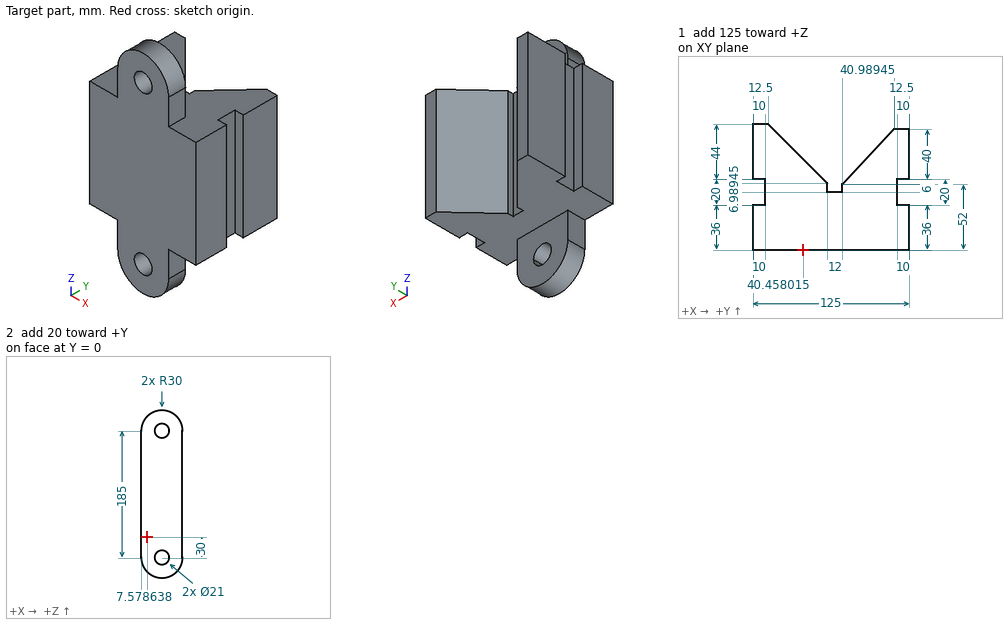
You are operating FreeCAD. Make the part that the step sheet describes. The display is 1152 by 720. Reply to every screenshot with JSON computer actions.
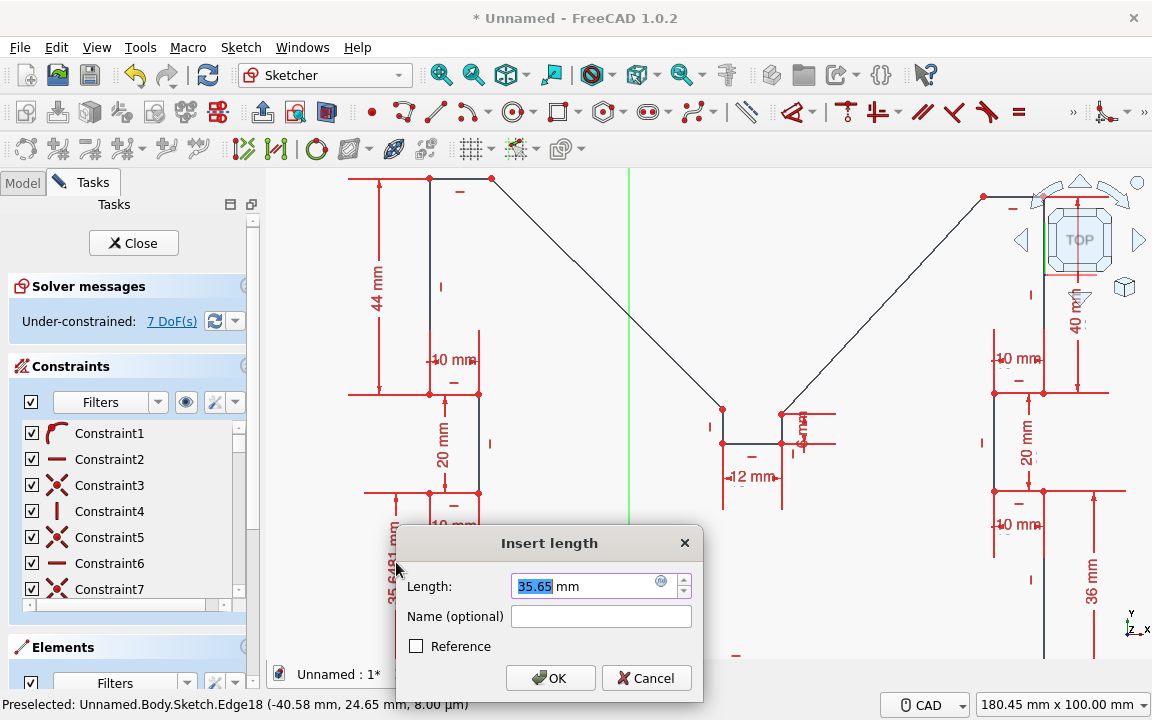
{"action": "type", "text": "36"}
{"action": "key", "text": "Return"}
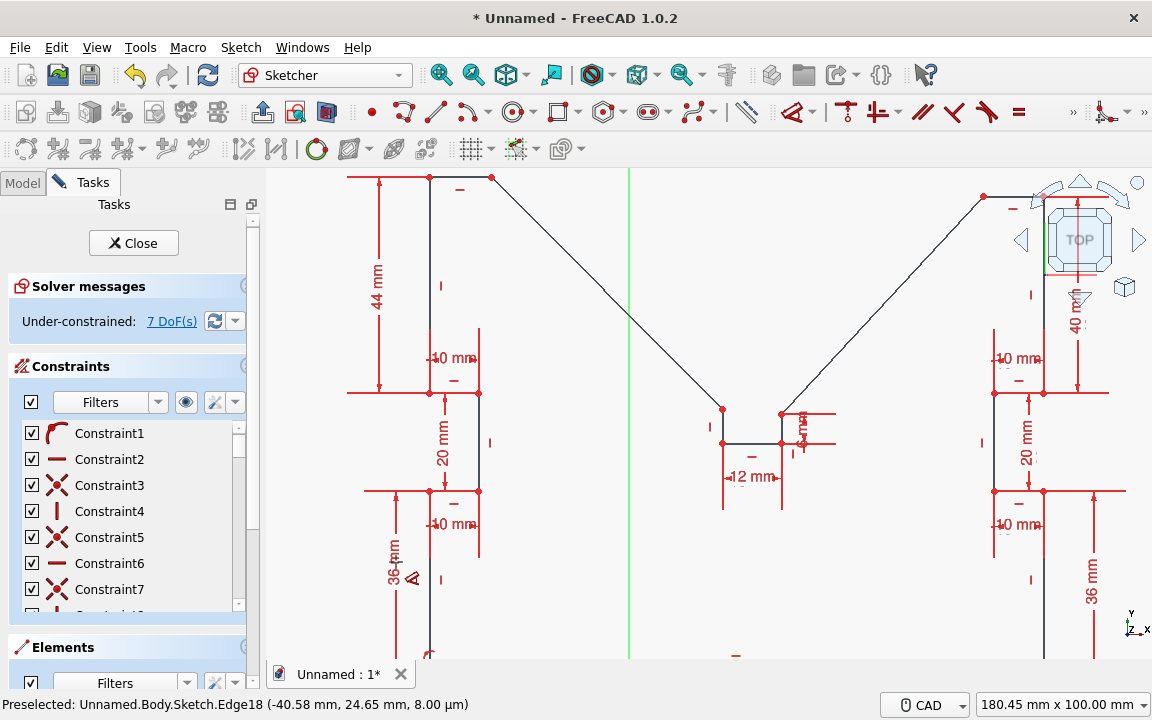
{"action": "scroll", "coordinate": [444, 395], "scroll_direction": "down", "scroll_amount": 2}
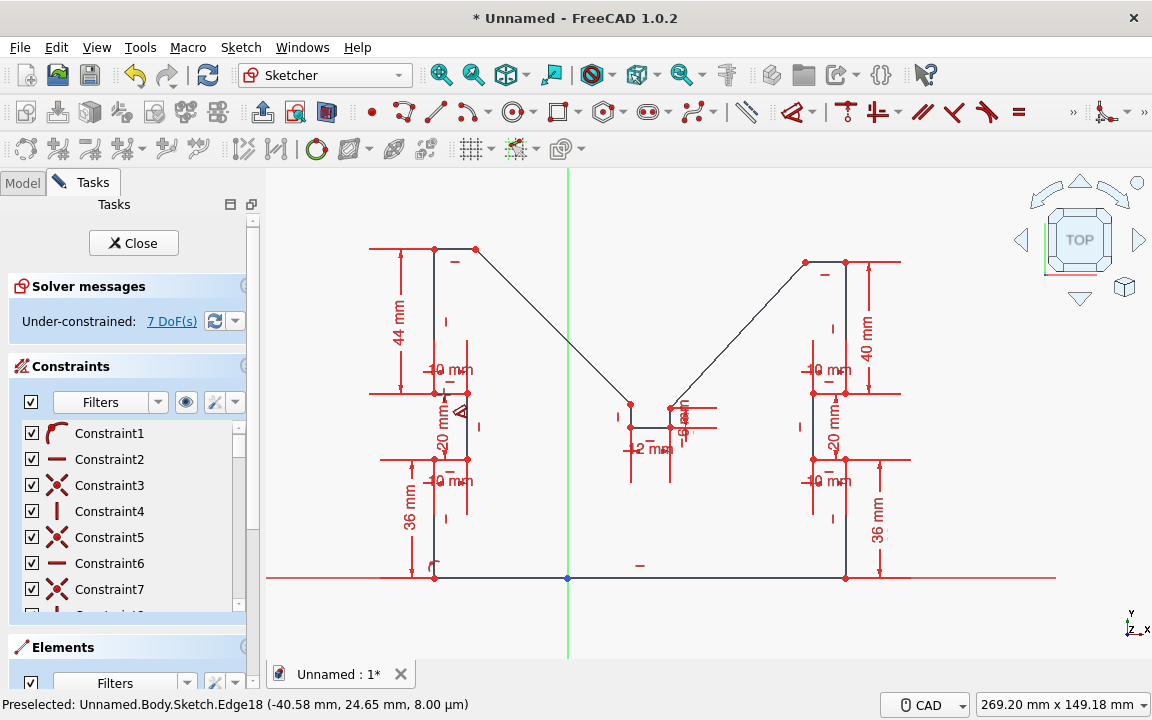
{"action": "scroll", "coordinate": [558, 578], "scroll_direction": "up", "scroll_amount": 2}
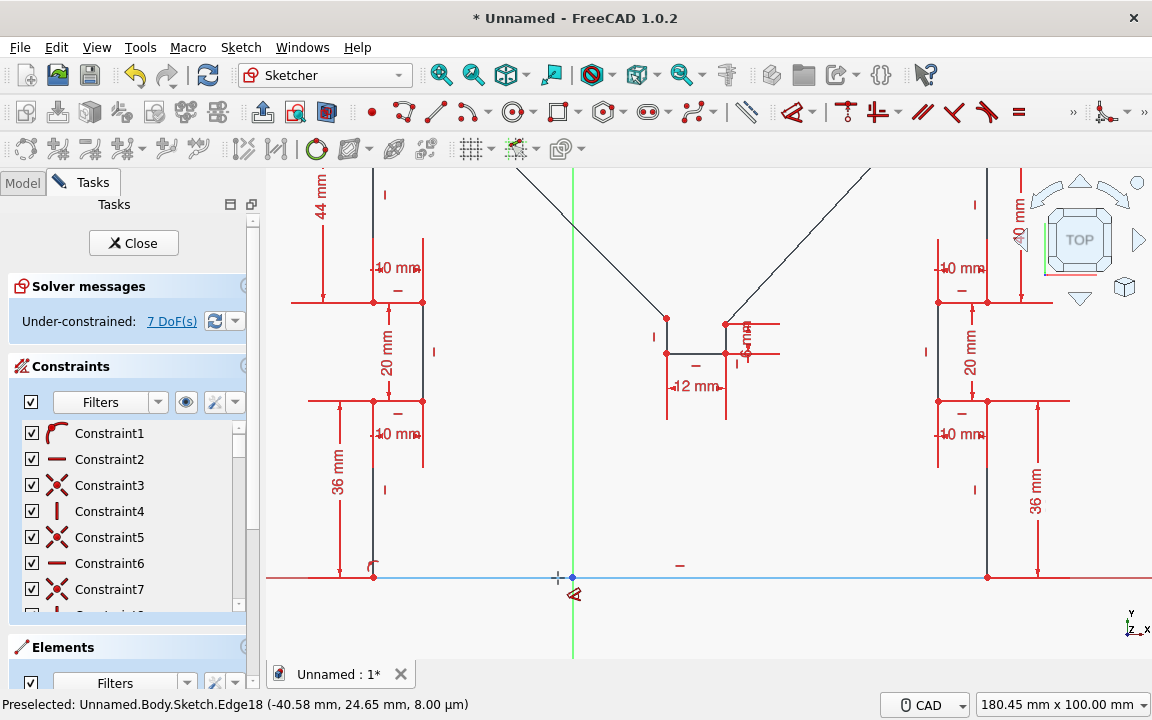
{"action": "left_click", "coordinate": [558, 578]}
{"action": "left_click", "coordinate": [680, 612]}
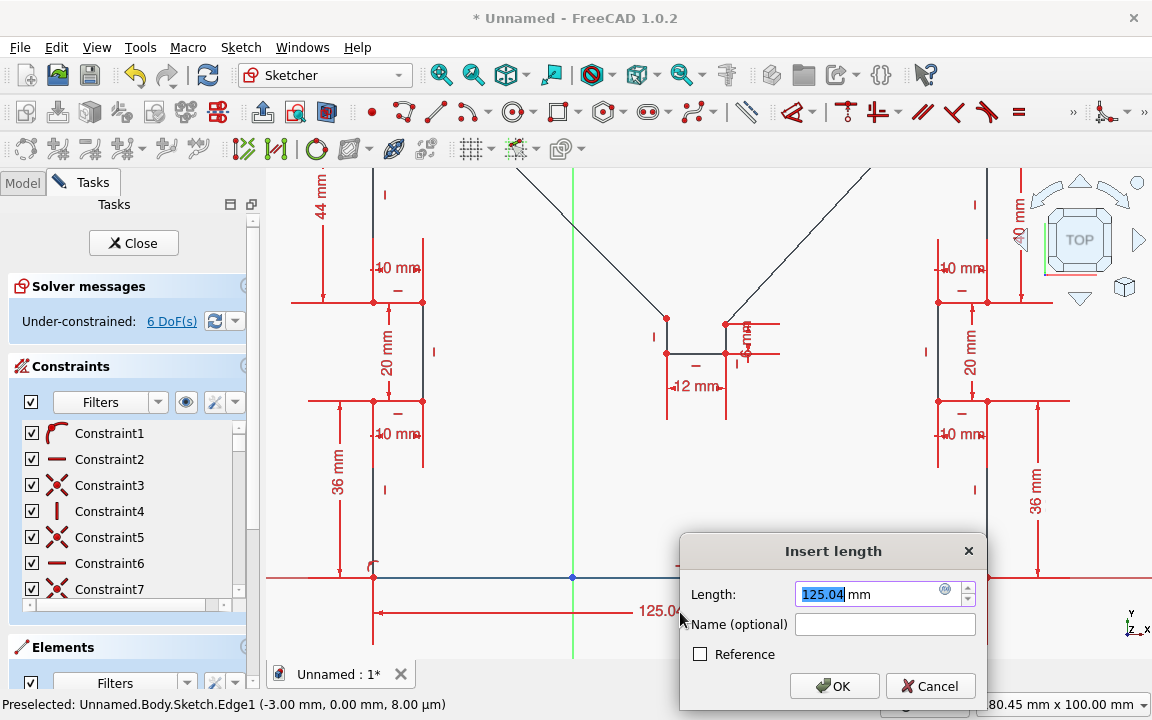
{"action": "type", "text": "125"}
{"action": "key", "text": "Return"}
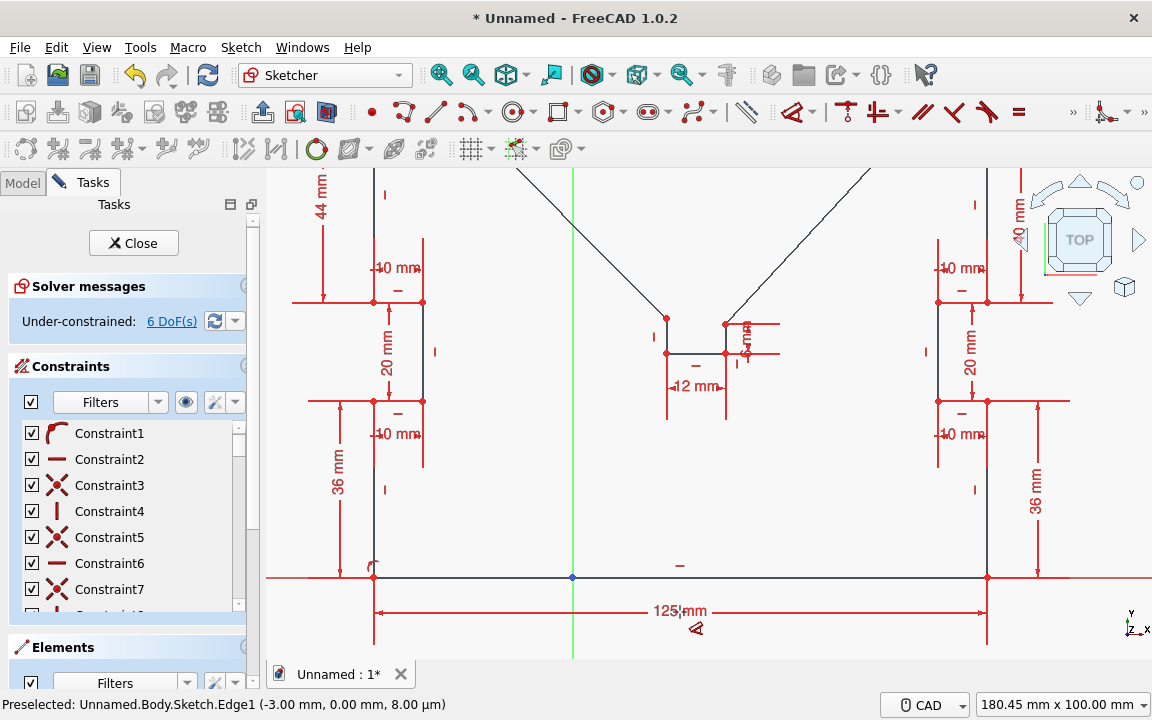
{"action": "left_click", "coordinate": [726, 324]}
{"action": "left_click", "coordinate": [539, 451]}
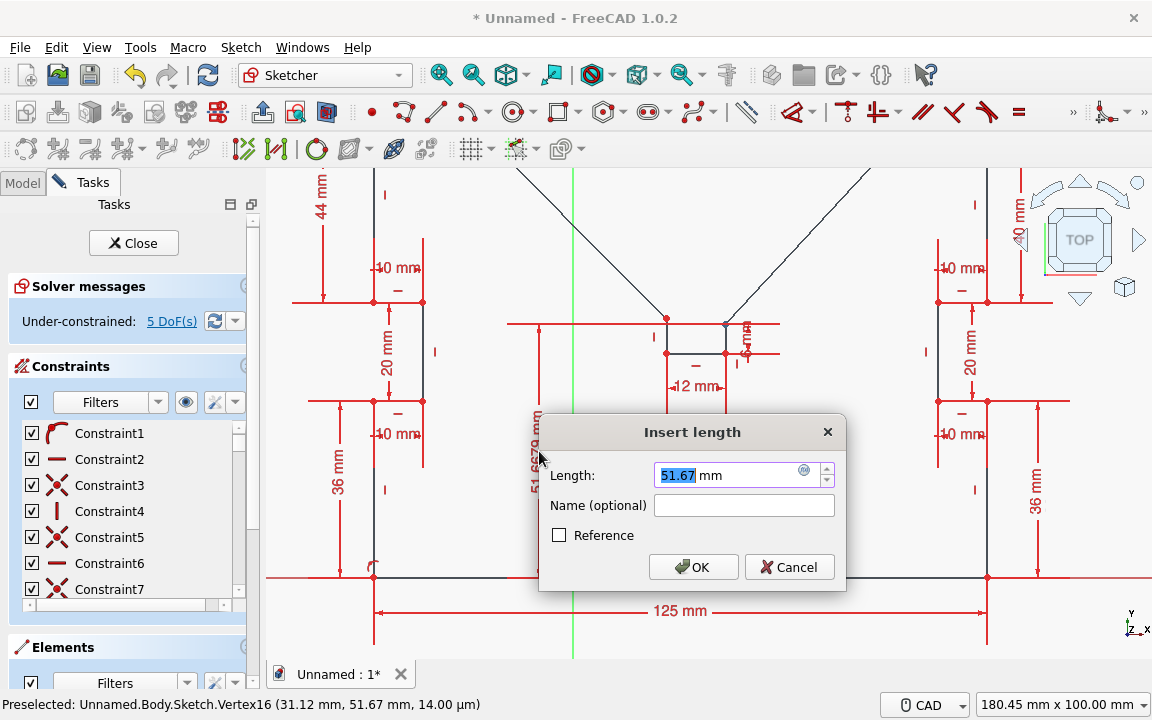
{"action": "type", "text": "52"}
{"action": "key", "text": "Return"}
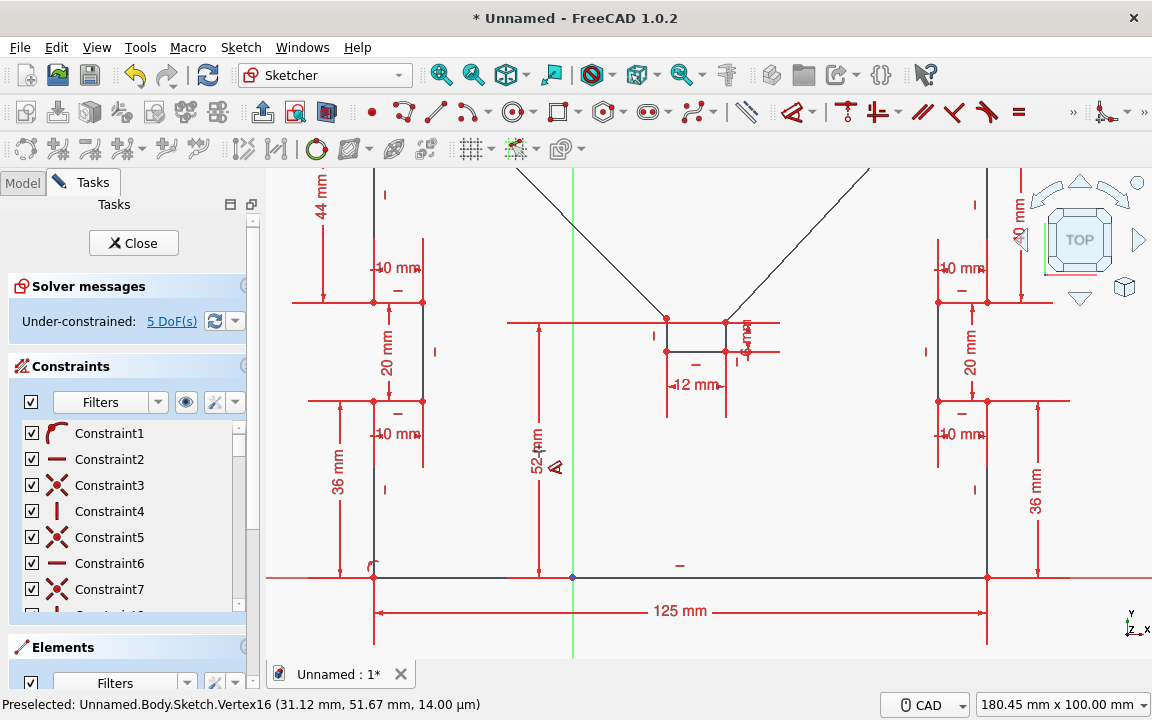
{"action": "scroll", "coordinate": [558, 579], "scroll_direction": "down", "scroll_amount": 2}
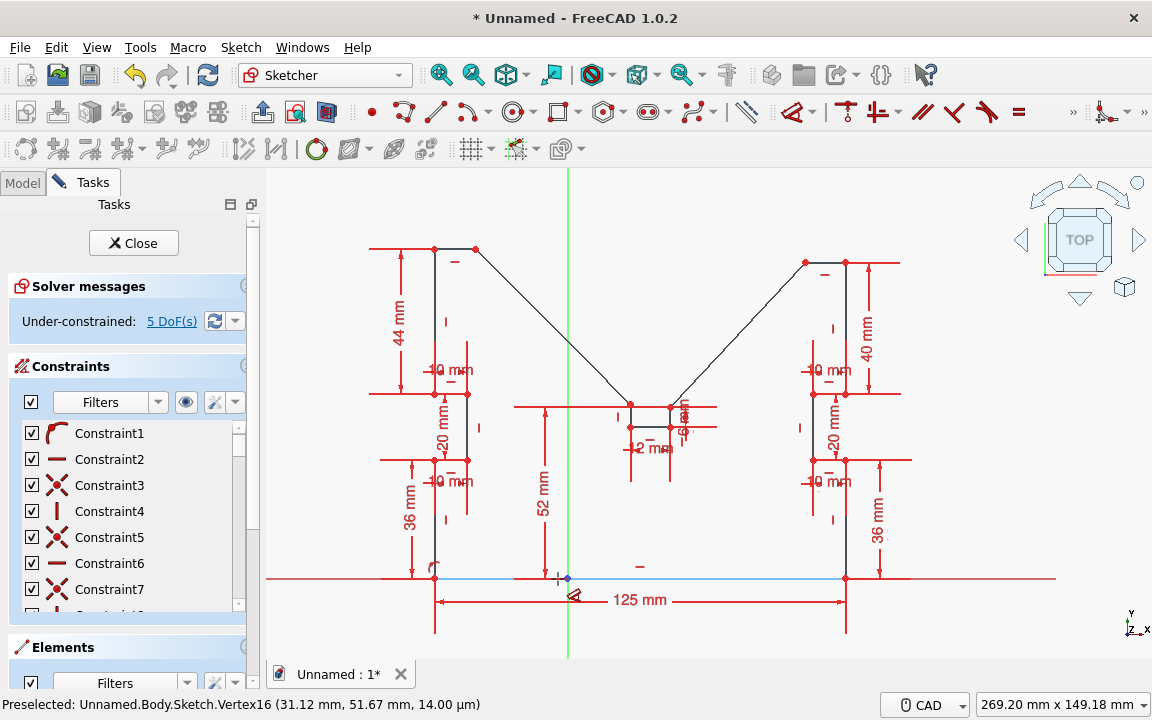
{"action": "left_click", "coordinate": [834, 263]}
{"action": "left_click", "coordinate": [826, 229]}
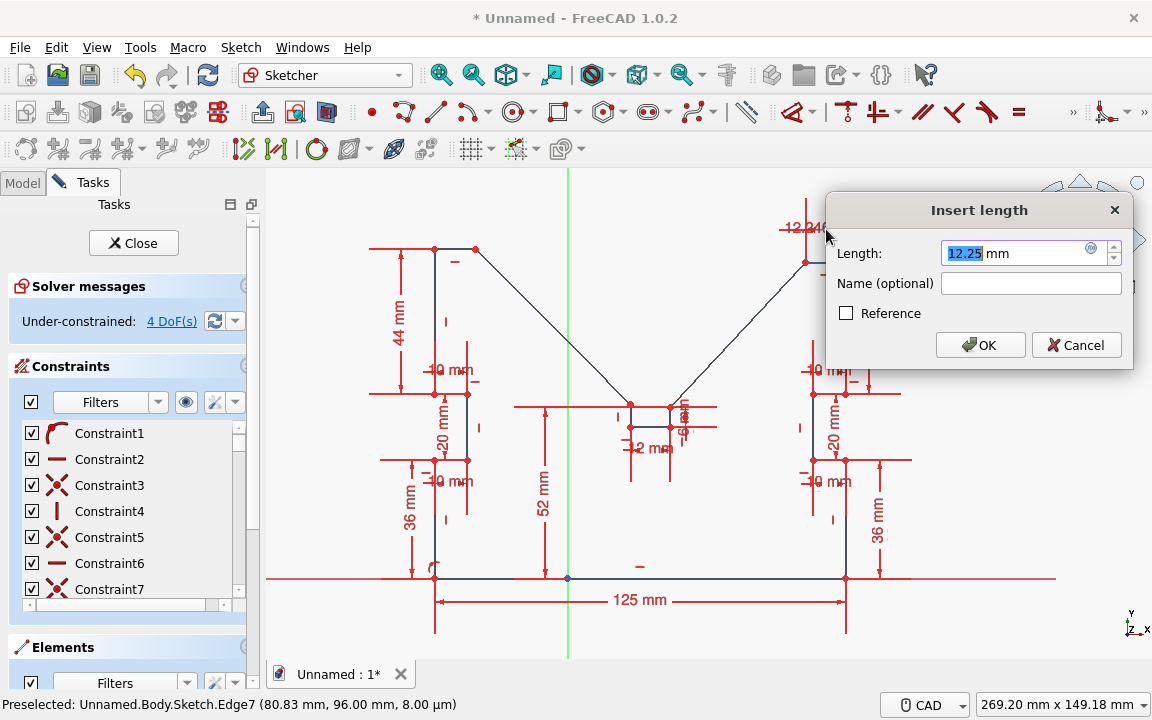
{"action": "type", "text": "12.5"}
{"action": "key", "text": "Return"}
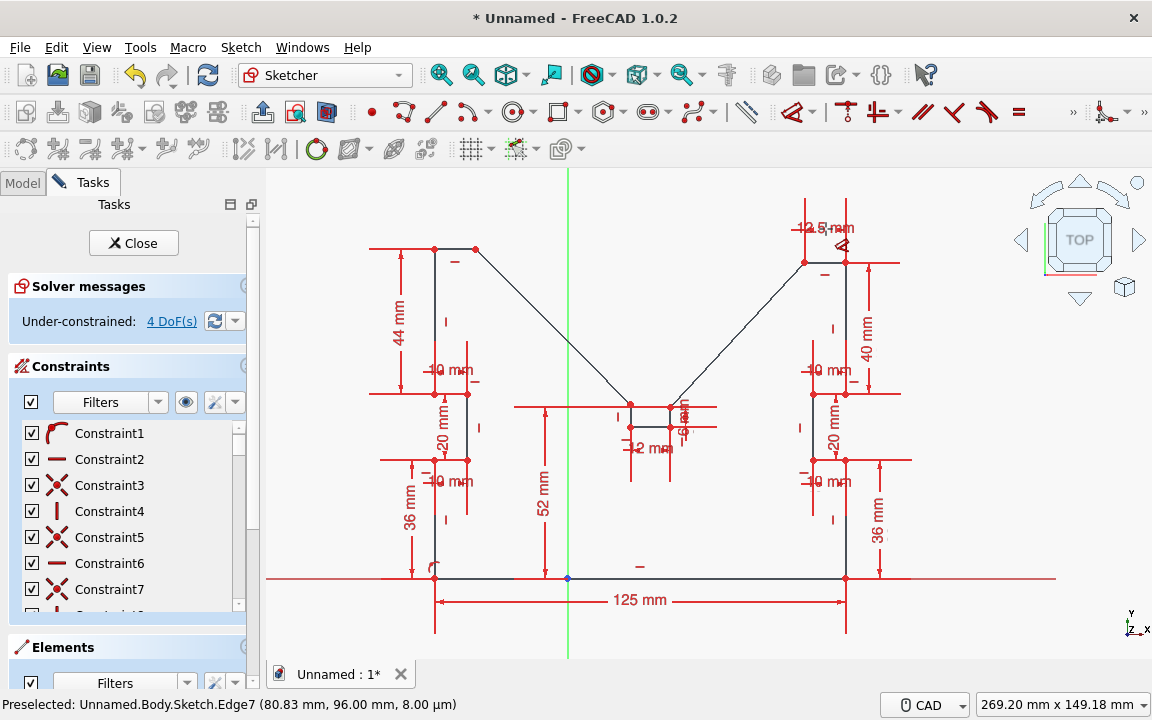
{"action": "left_click", "coordinate": [463, 249]}
{"action": "left_click", "coordinate": [455, 215]}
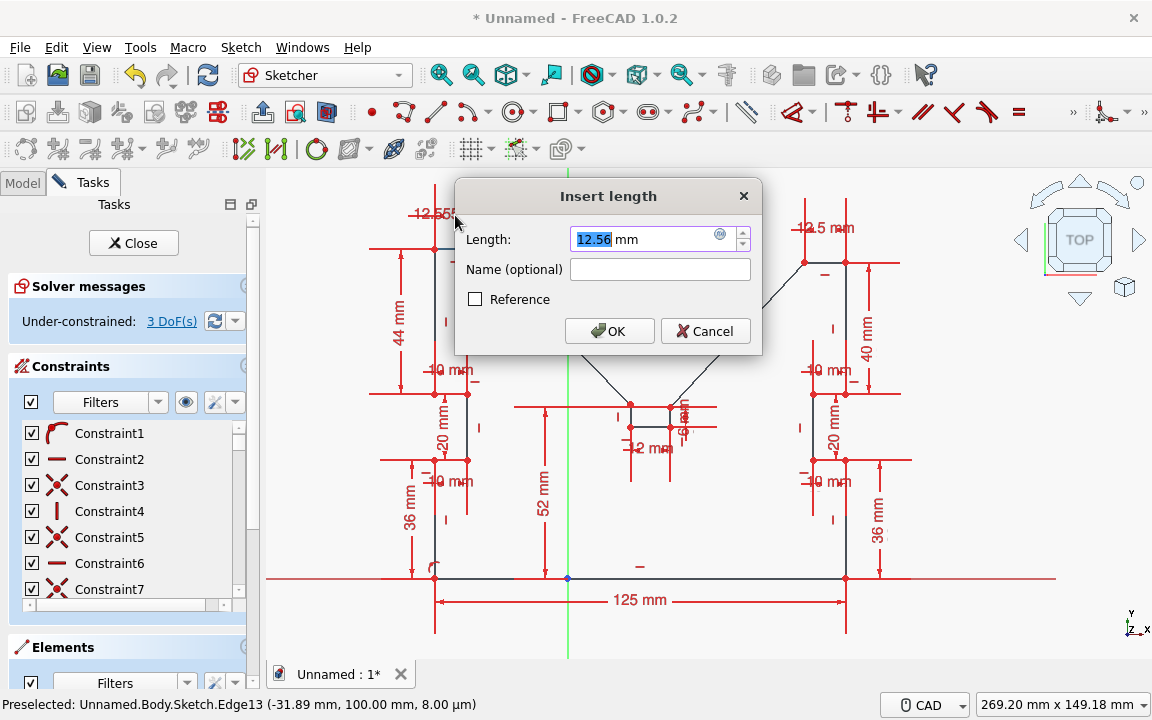
{"action": "type", "text": "12.5"}
{"action": "key", "text": "Return"}